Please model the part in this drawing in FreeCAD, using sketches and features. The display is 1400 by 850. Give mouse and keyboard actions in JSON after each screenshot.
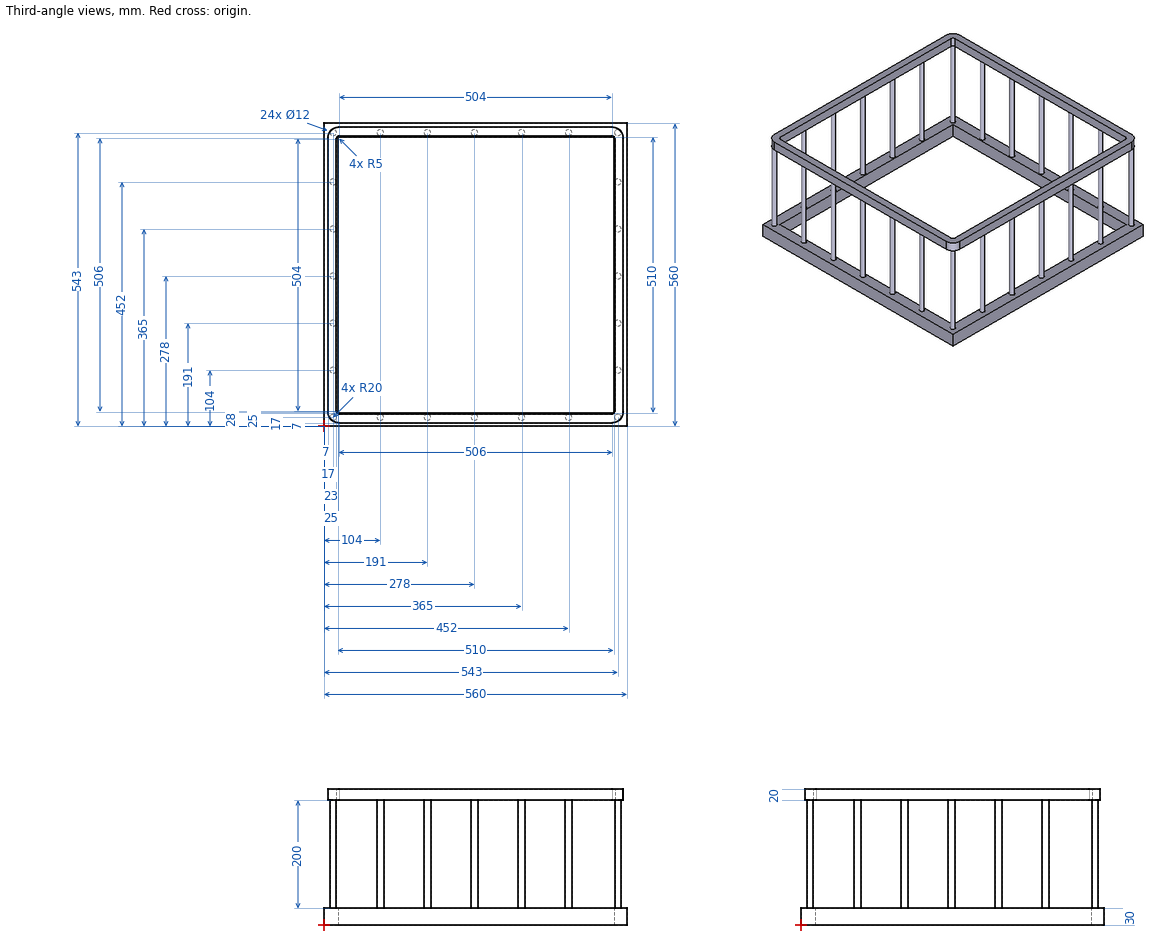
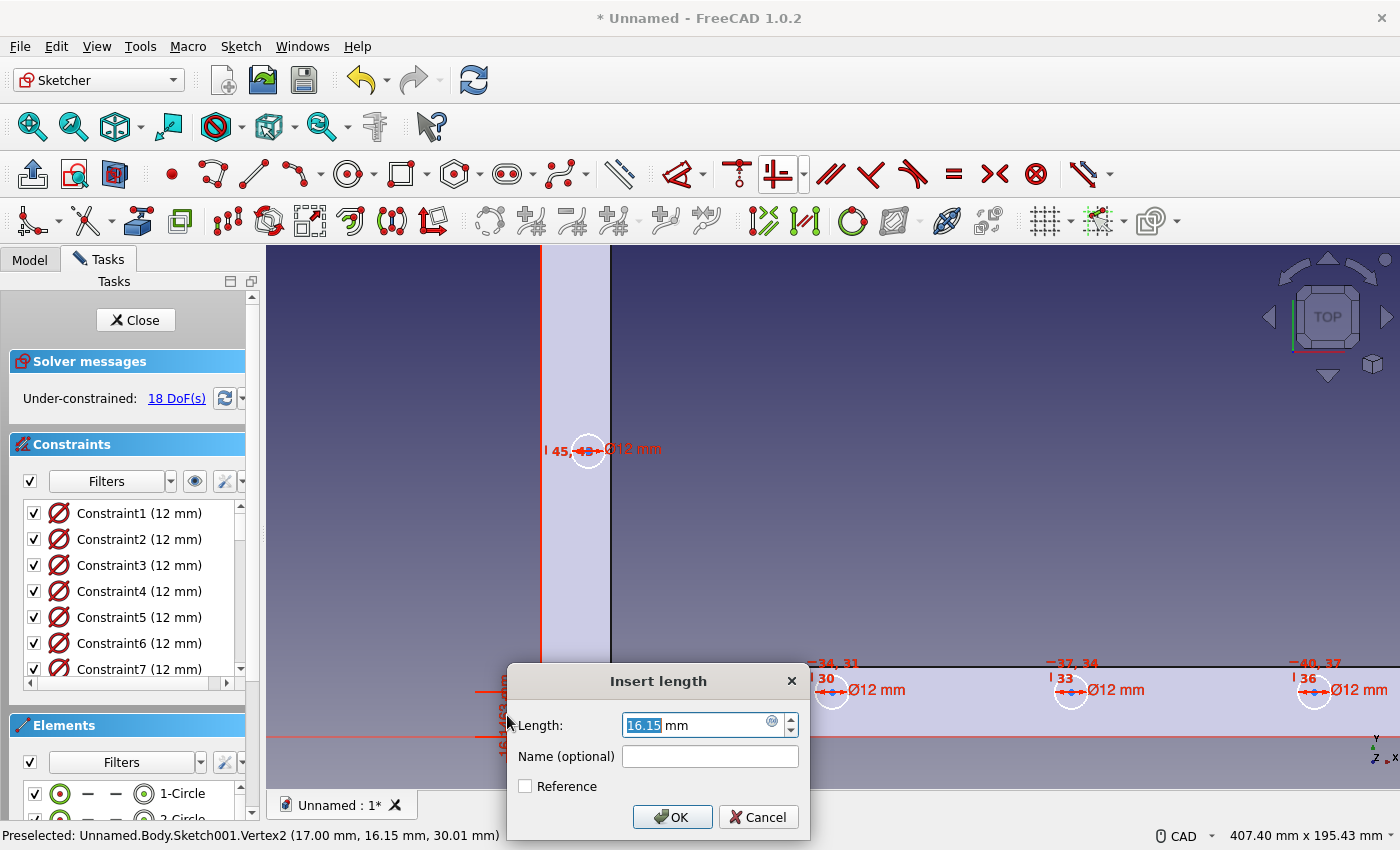
{"action": "type", "text": "17"}
{"action": "key", "text": "Return"}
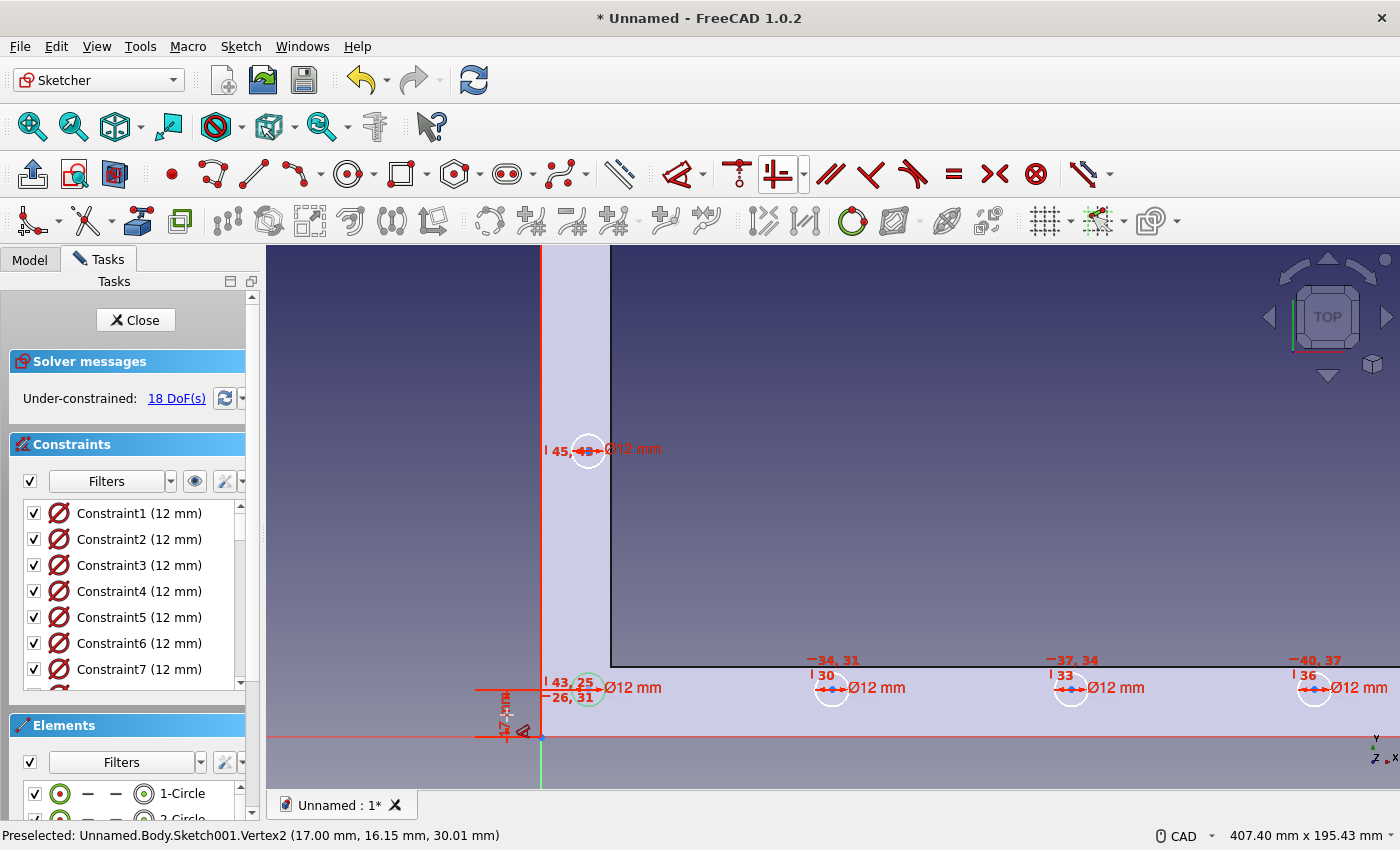
{"action": "scroll", "coordinate": [588, 695], "scroll_direction": "down", "scroll_amount": 7}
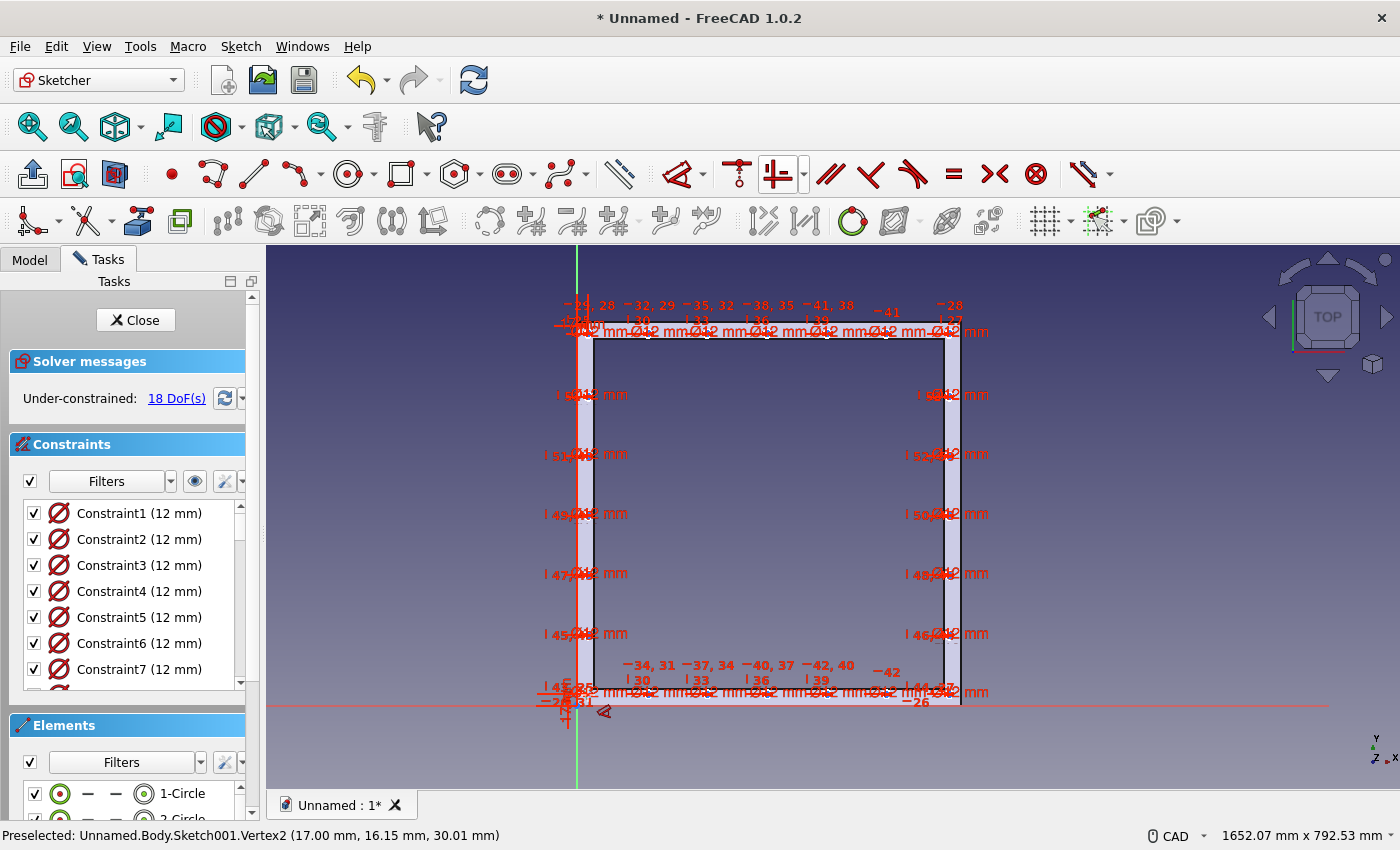
{"action": "left_click", "coordinate": [588, 334]}
{"action": "left_click", "coordinate": [543, 520]}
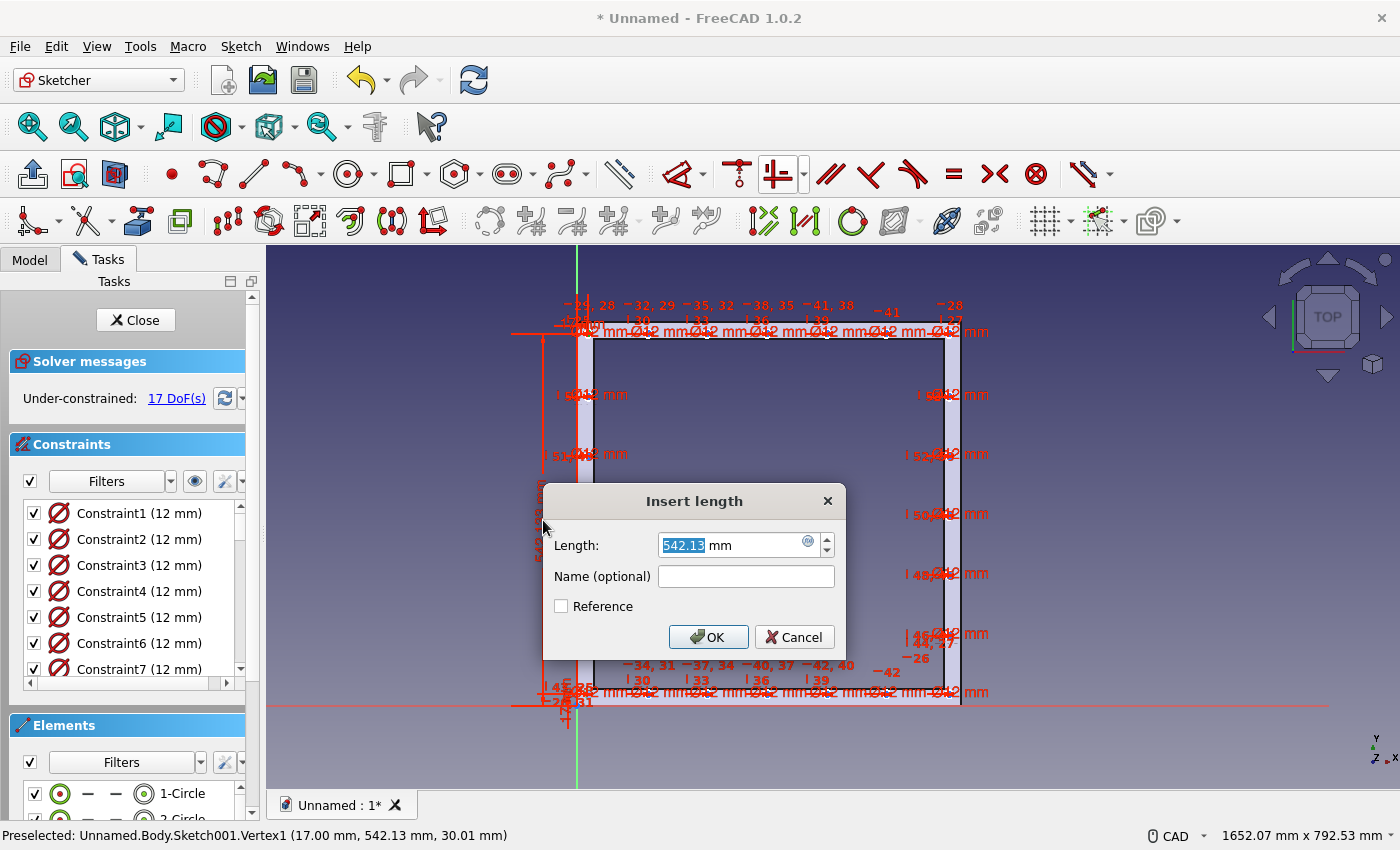
{"action": "type", "text": "543"}
{"action": "key", "text": "Return"}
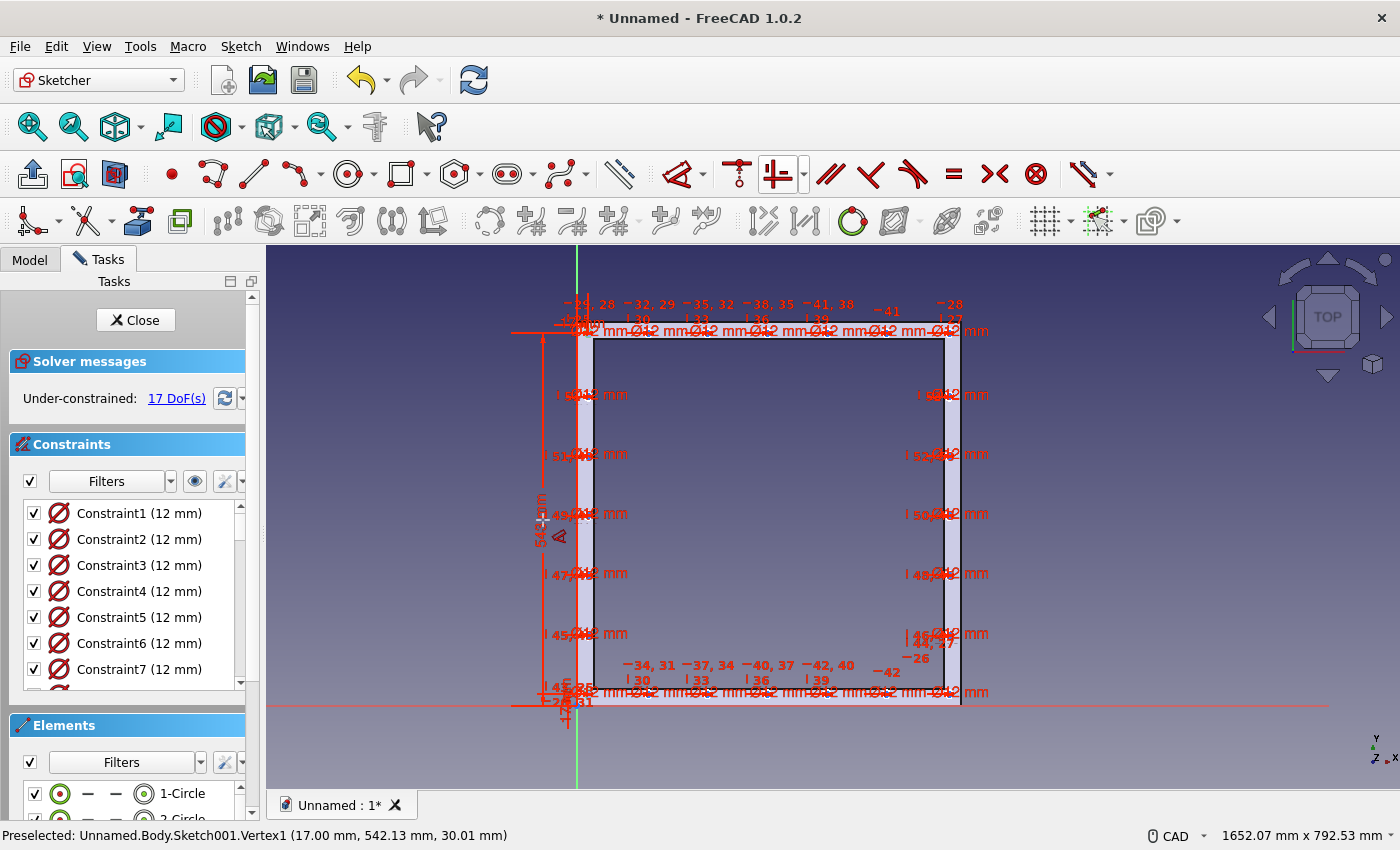
{"action": "left_click", "coordinate": [949, 694]}
{"action": "left_click", "coordinate": [763, 740]}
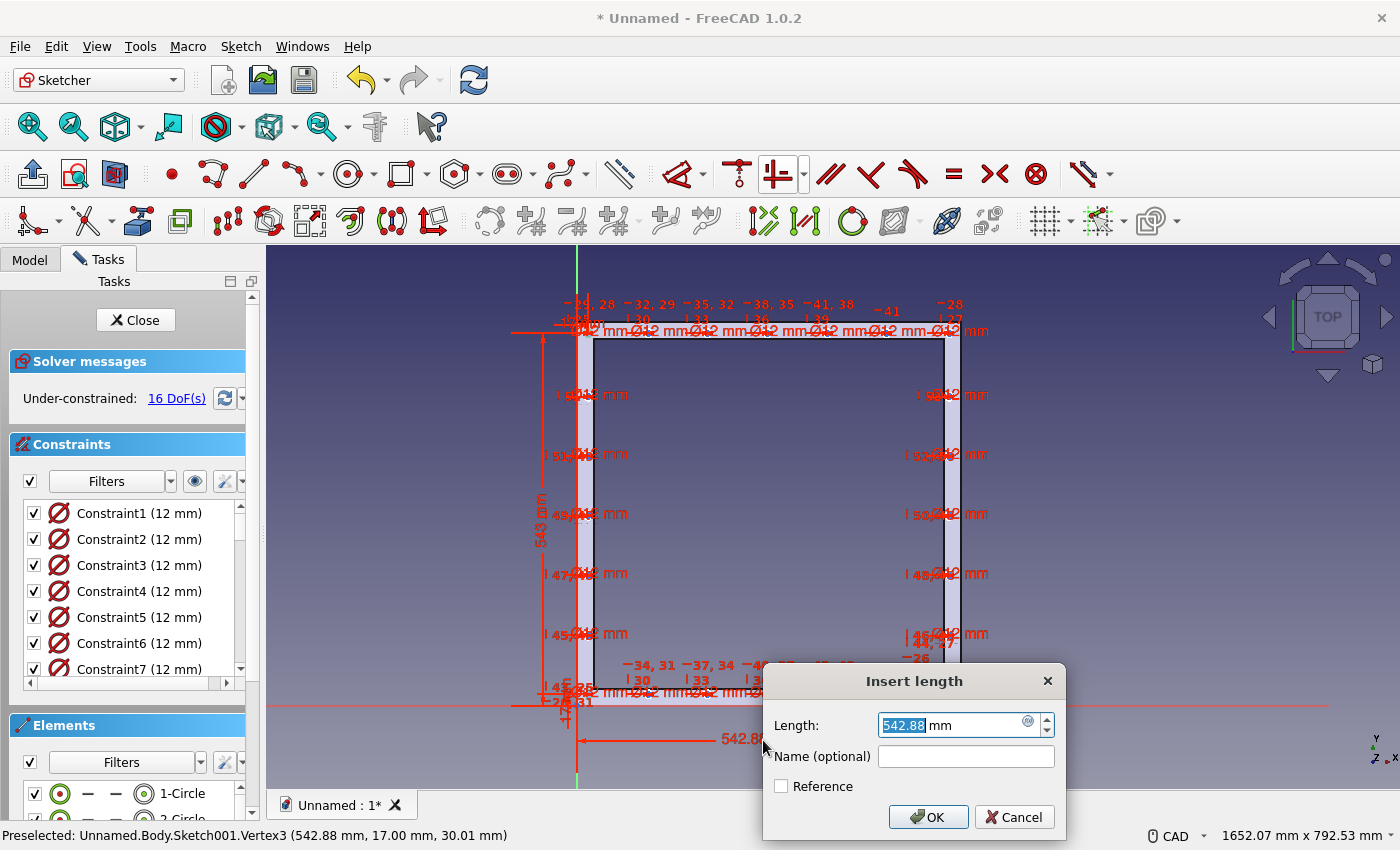
{"action": "type", "text": "543"}
{"action": "key", "text": "Return"}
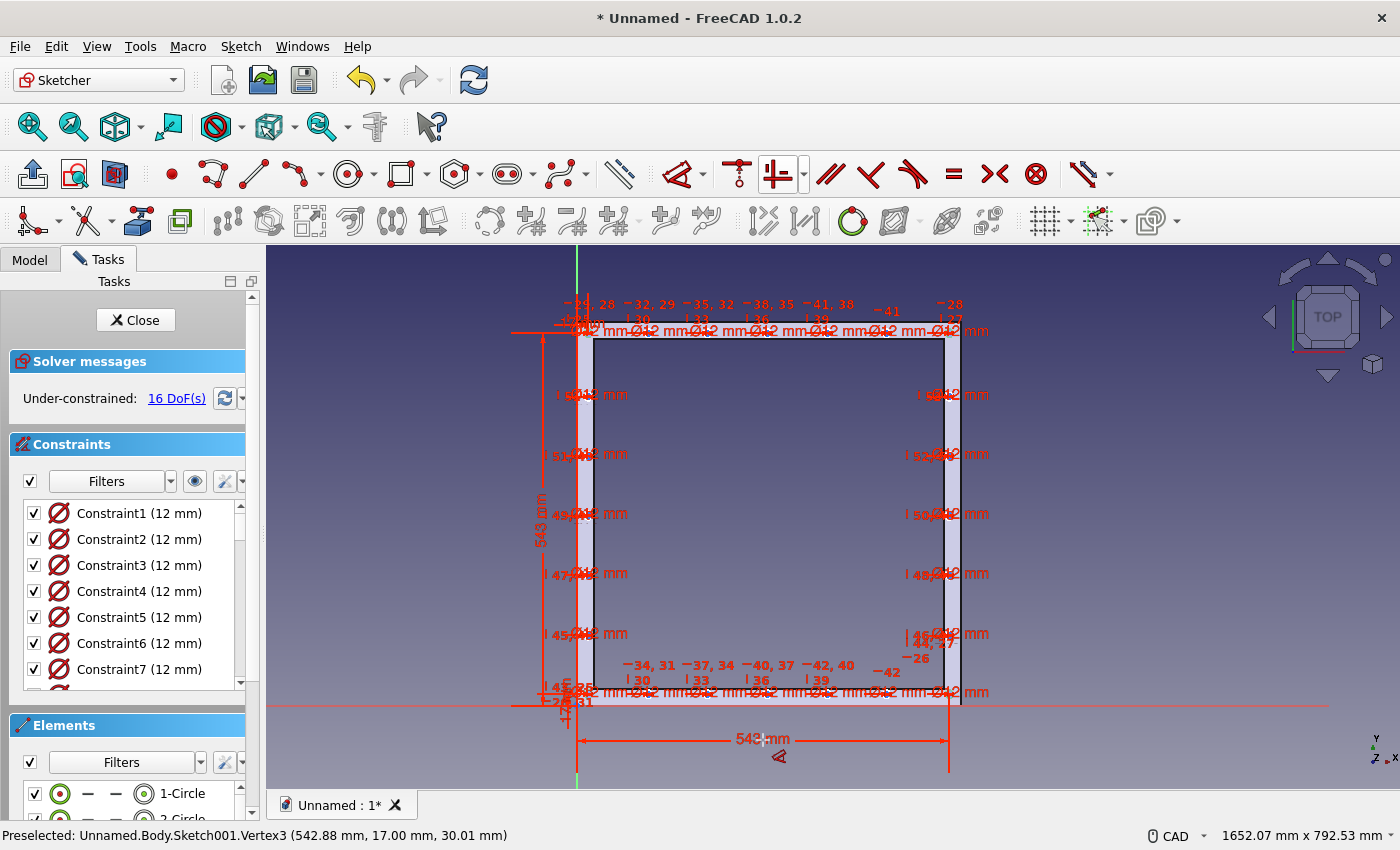
{"action": "left_click", "coordinate": [648, 333]}
{"action": "left_click", "coordinate": [613, 740]}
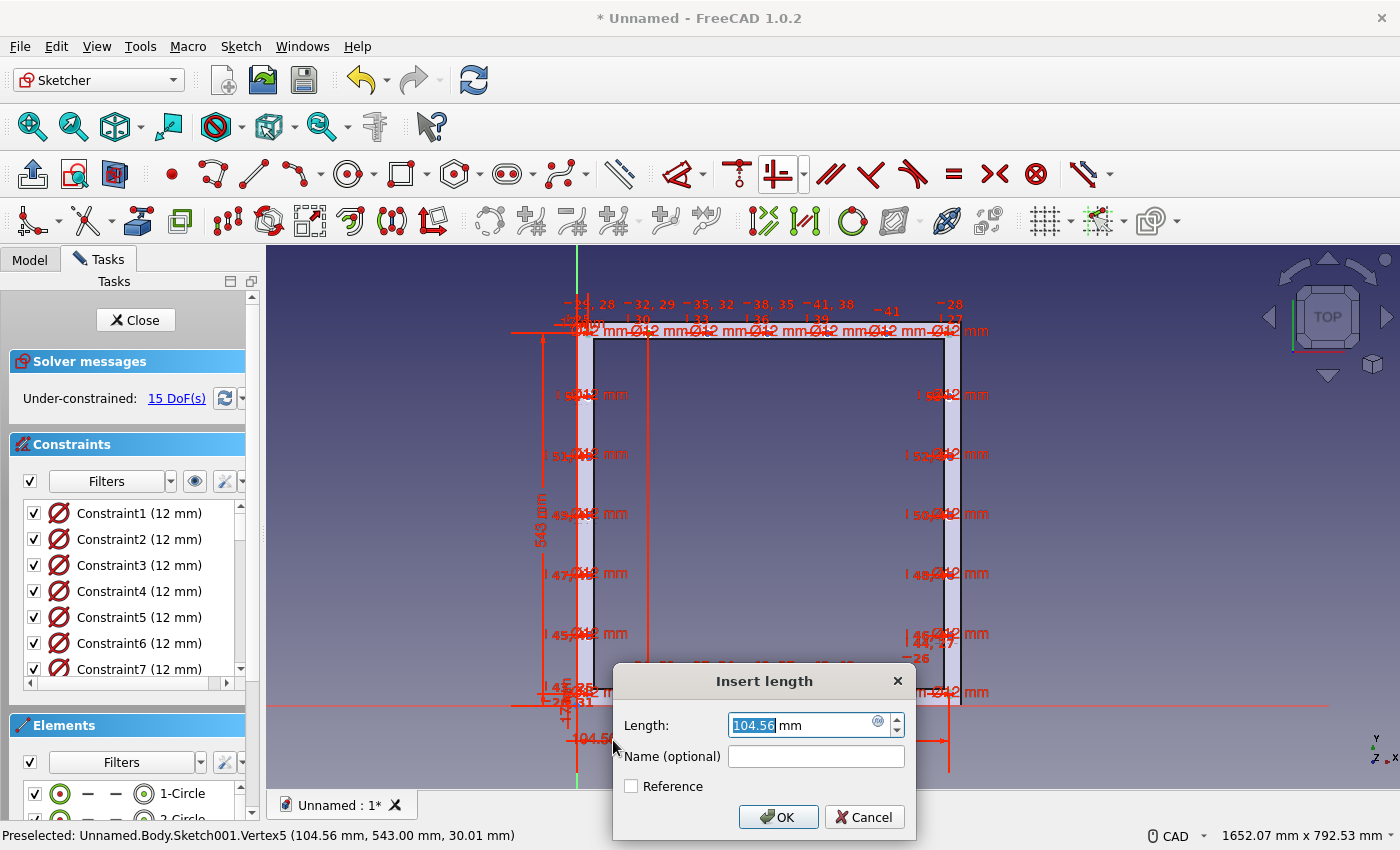
{"action": "type", "text": "104"}
{"action": "key", "text": "Return"}